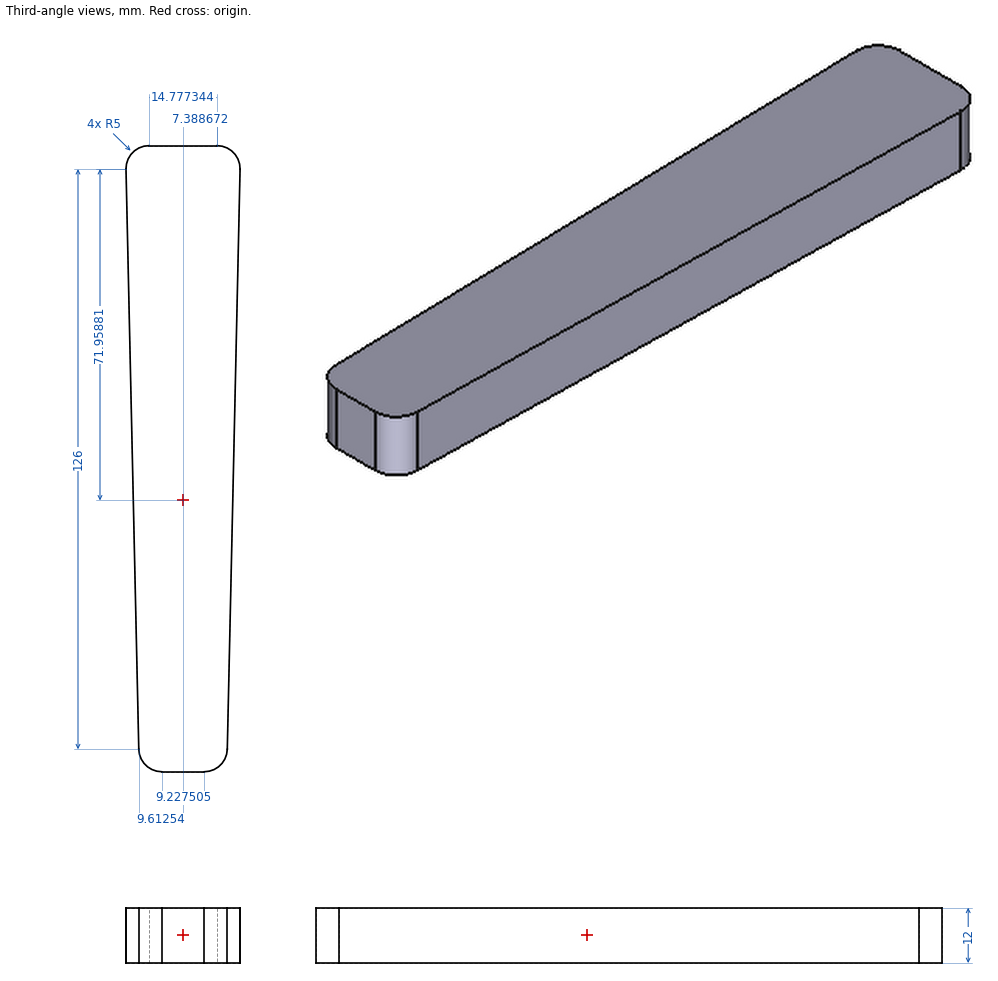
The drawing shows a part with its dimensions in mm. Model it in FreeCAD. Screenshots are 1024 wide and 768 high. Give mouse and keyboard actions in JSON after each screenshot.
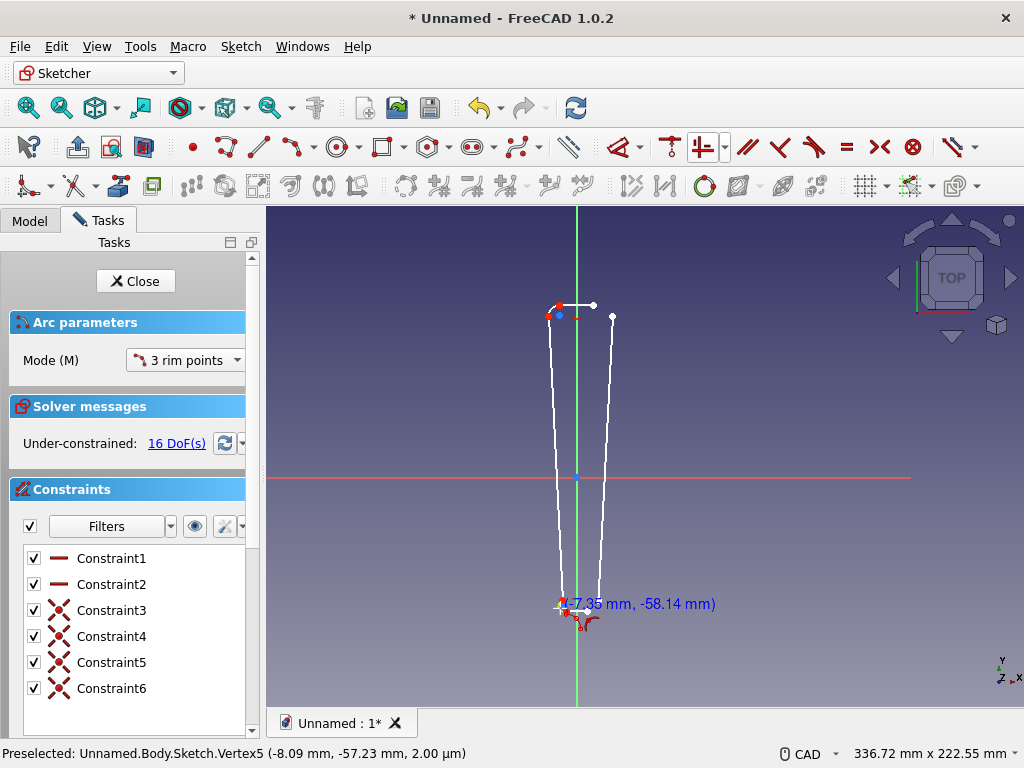
{"action": "scroll", "coordinate": [587, 611], "scroll_direction": "up", "scroll_amount": 3}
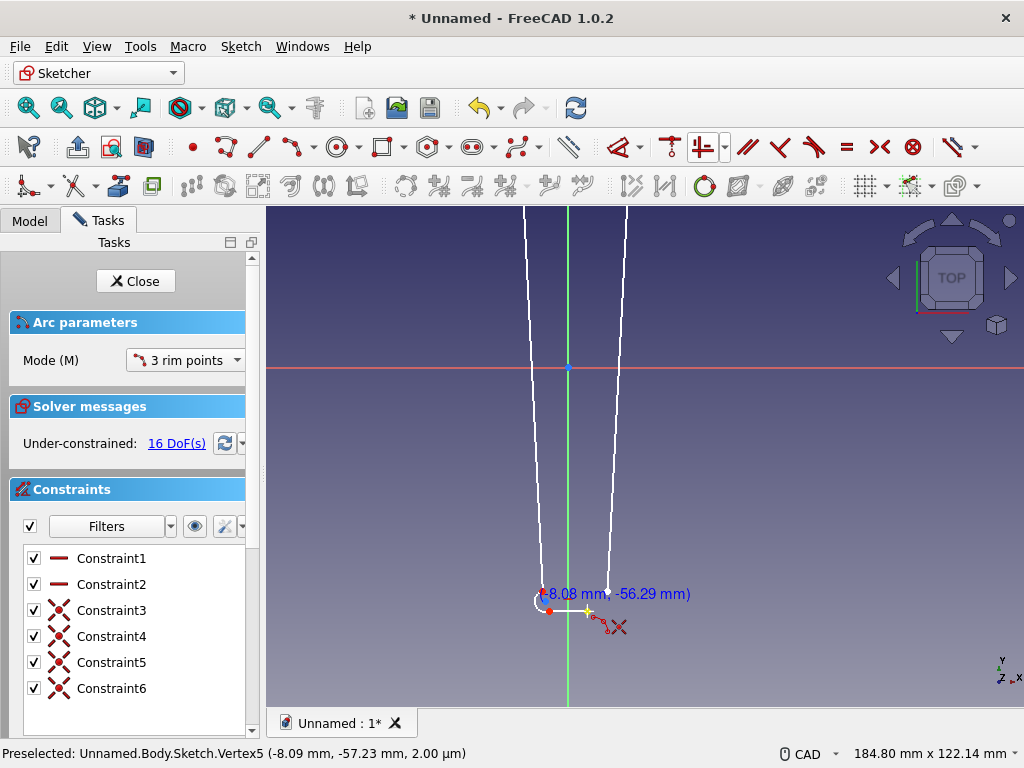
{"action": "left_click", "coordinate": [587, 611]}
{"action": "left_click", "coordinate": [607, 591]}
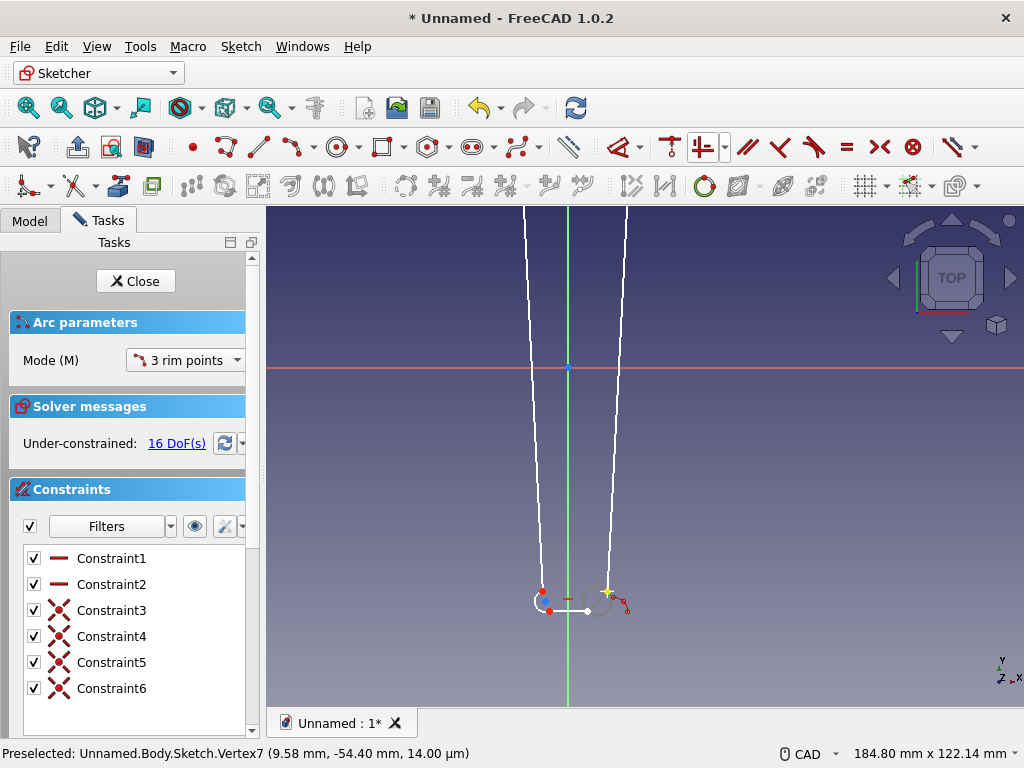
{"action": "scroll", "coordinate": [601, 604], "scroll_direction": "up", "scroll_amount": 5}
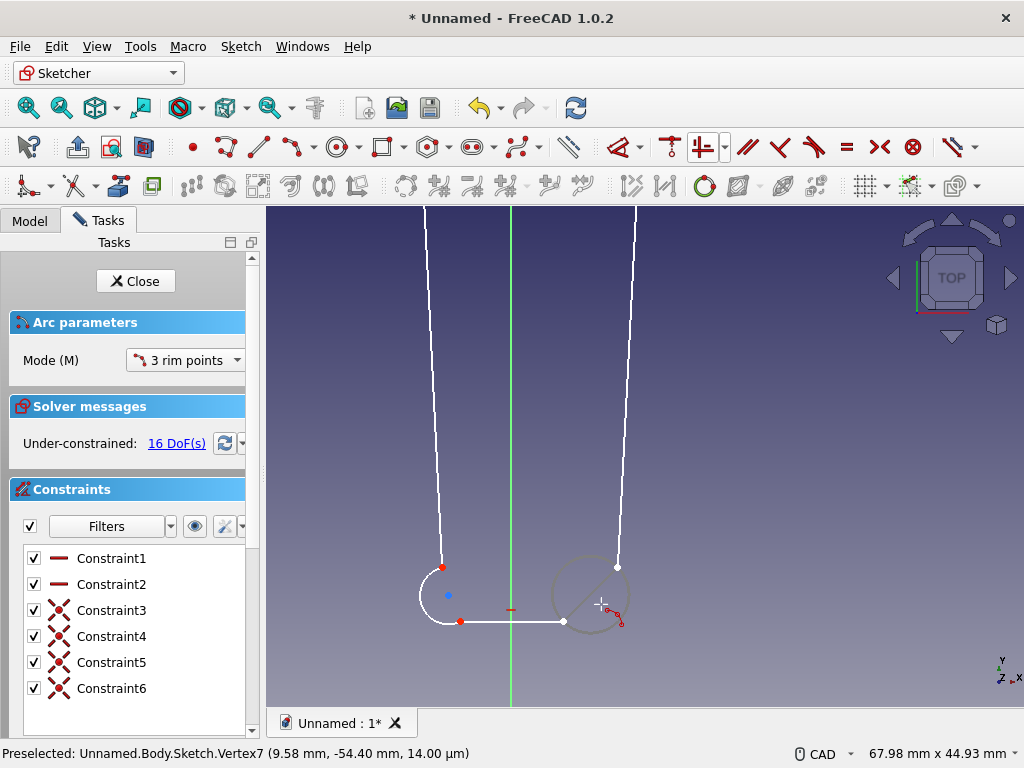
{"action": "left_click", "coordinate": [601, 602]}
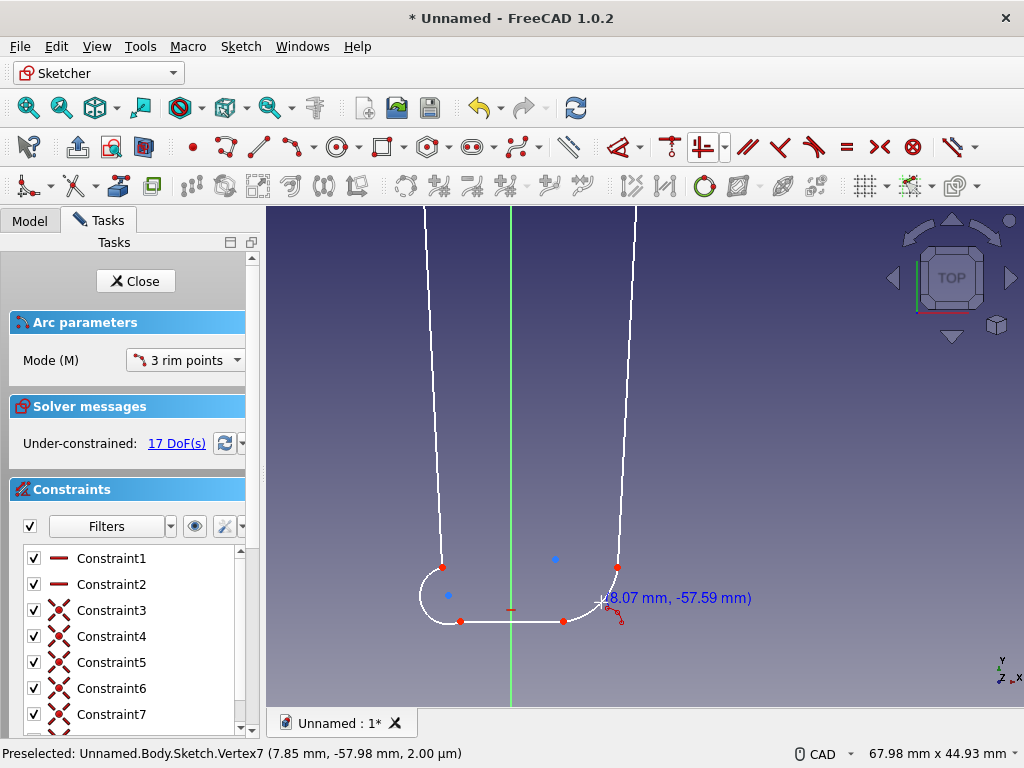
{"action": "scroll", "coordinate": [593, 607], "scroll_direction": "down", "scroll_amount": 8}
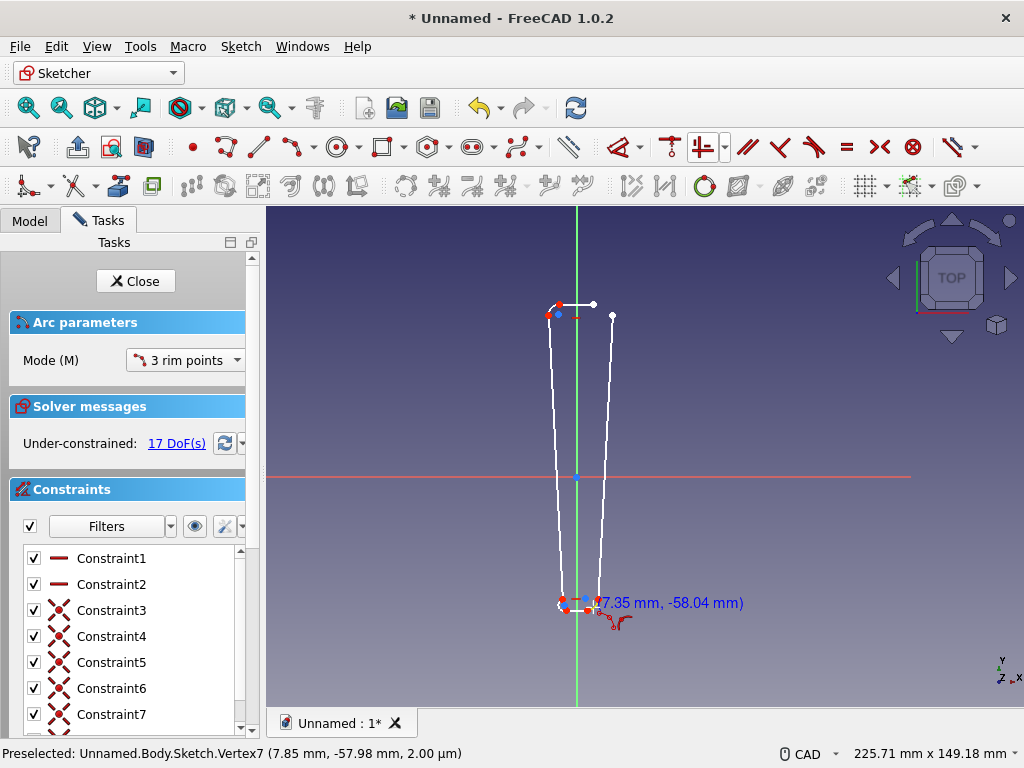
{"action": "left_click", "coordinate": [613, 316]}
{"action": "left_click", "coordinate": [594, 305]}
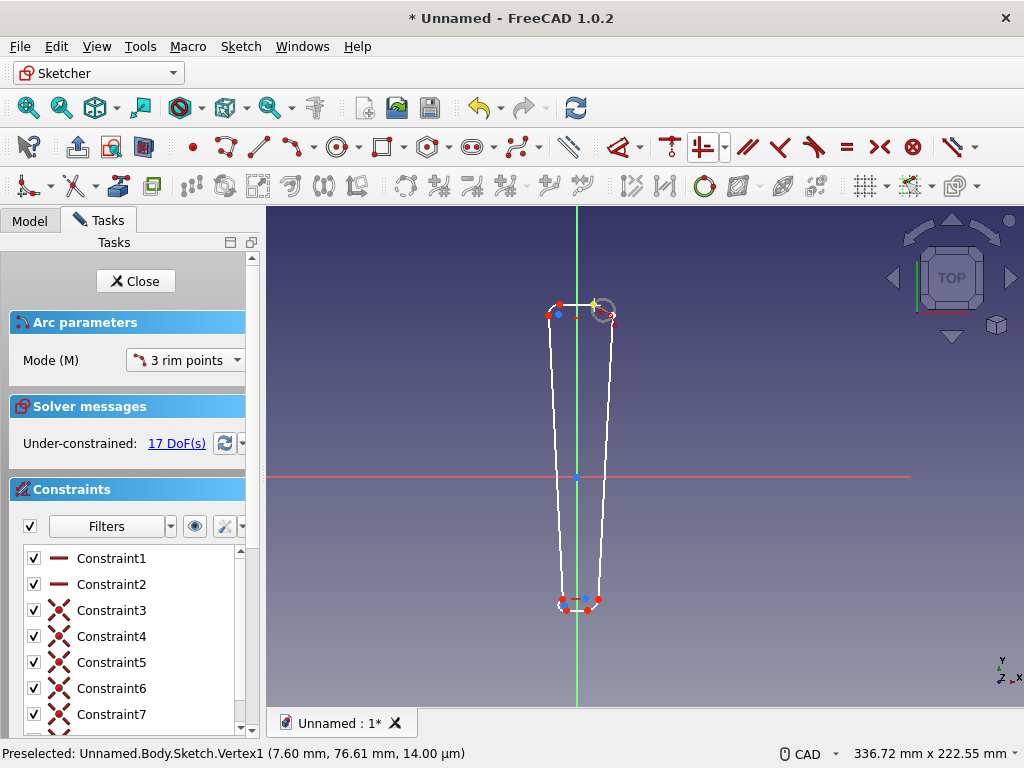
{"action": "scroll", "coordinate": [601, 307], "scroll_direction": "up", "scroll_amount": 8}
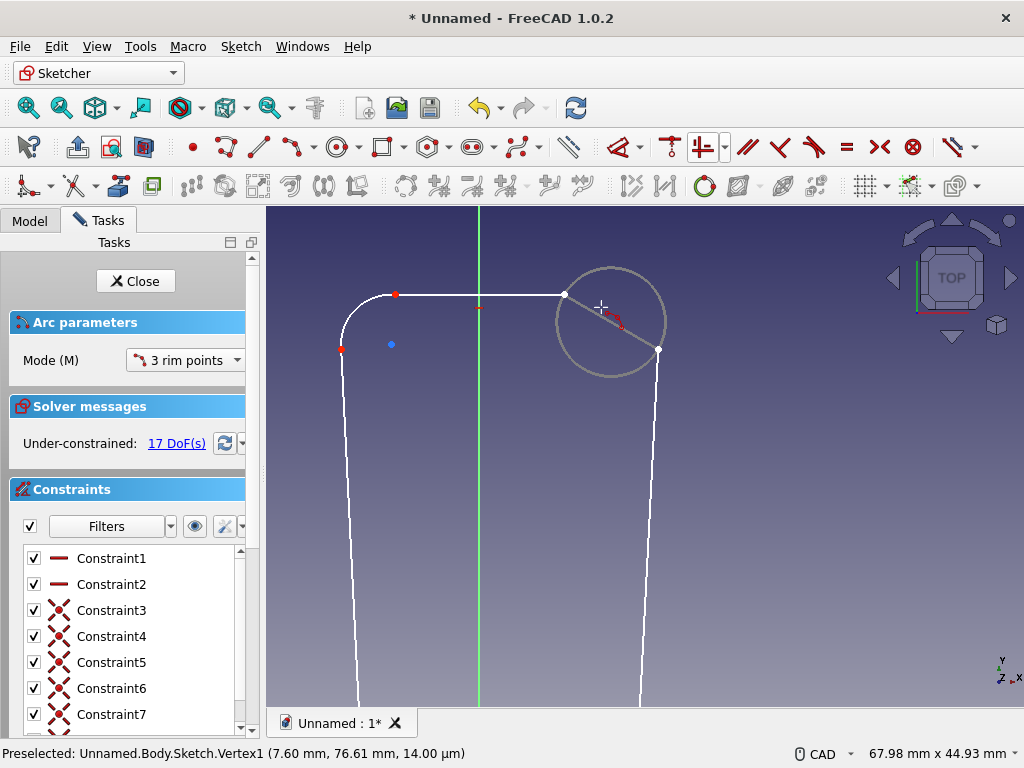
{"action": "left_click", "coordinate": [602, 307]}
{"action": "key", "text": "Escape"}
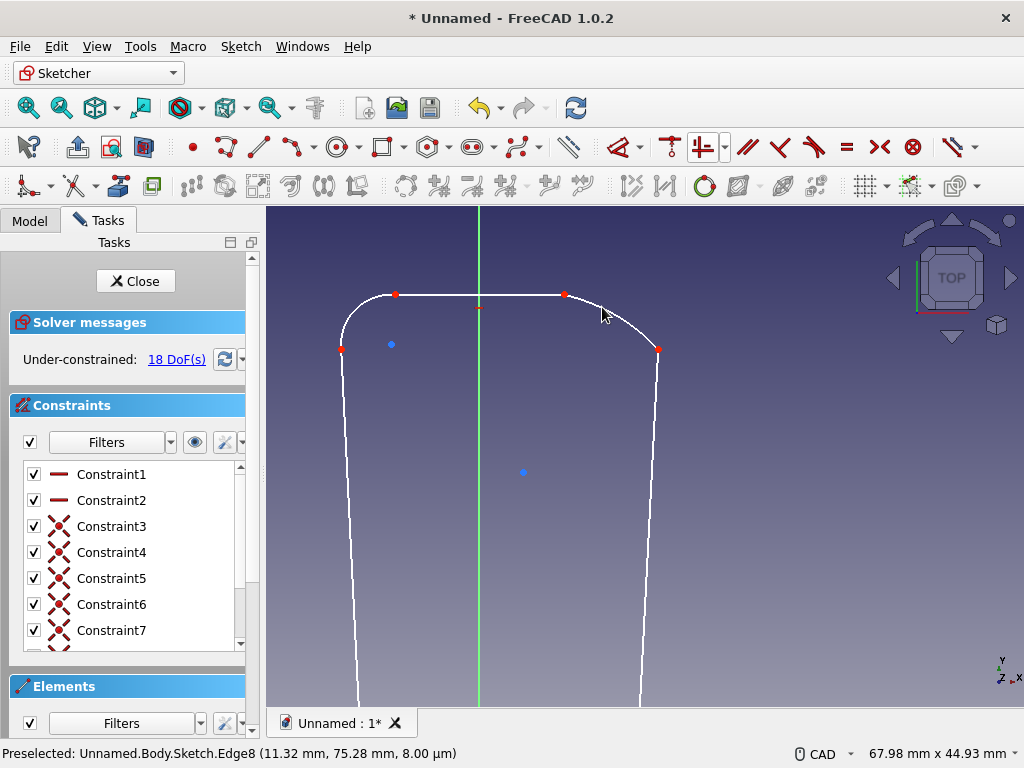
{"action": "left_click", "coordinate": [514, 295]}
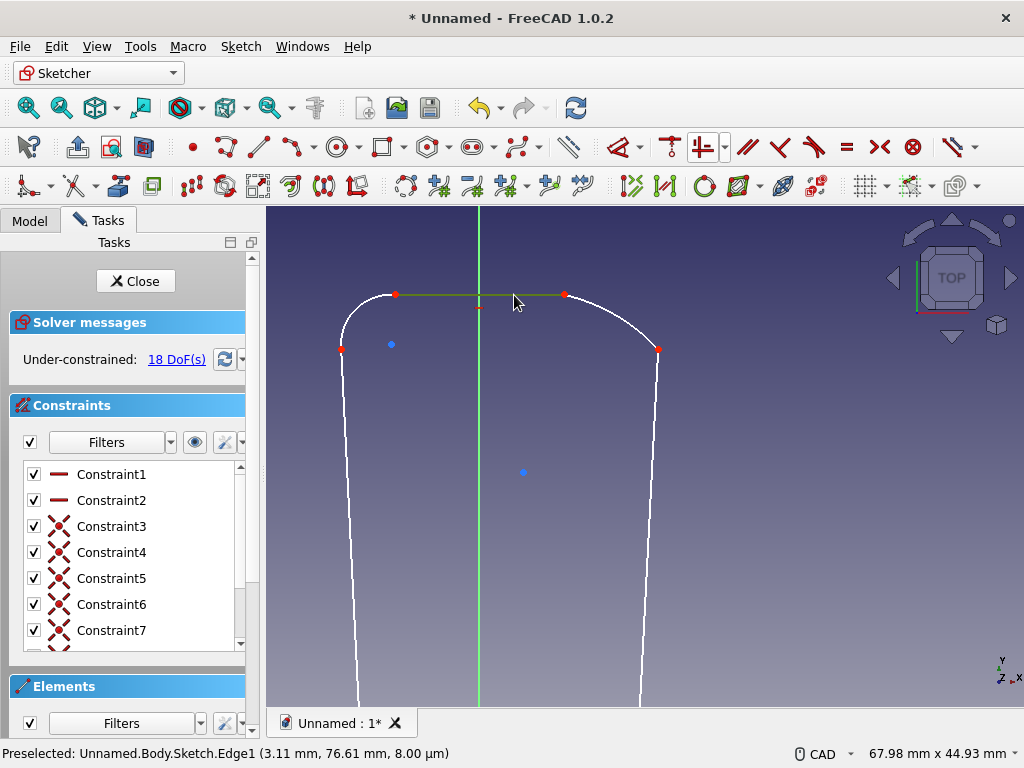
{"action": "left_click", "coordinate": [370, 299]}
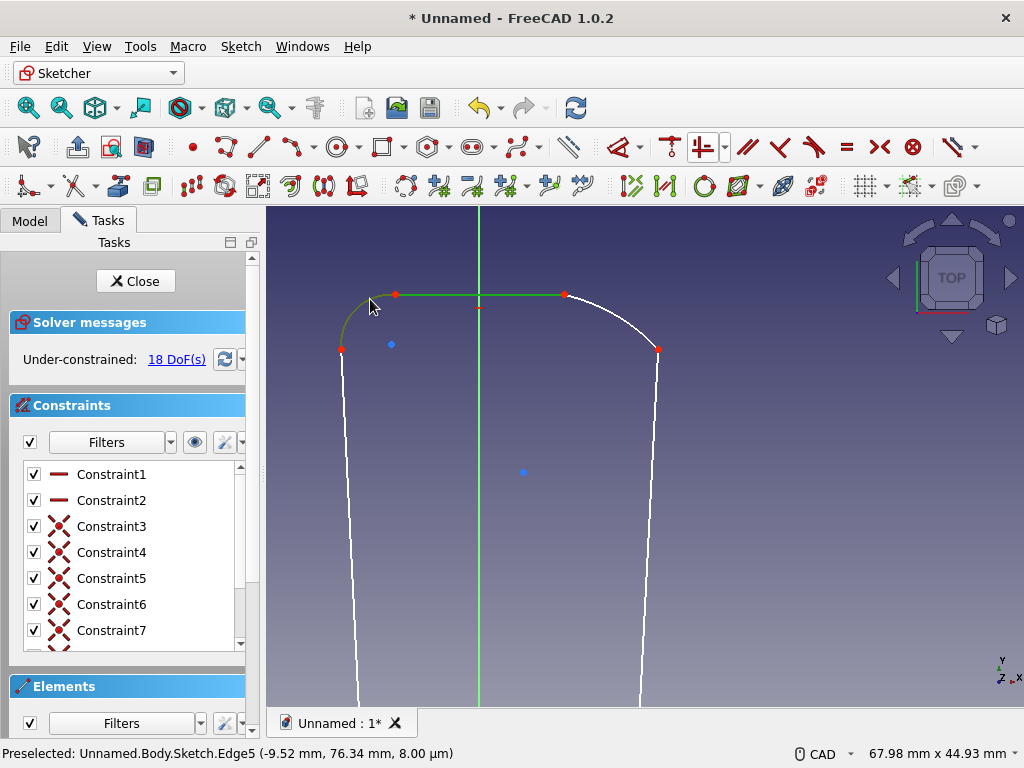
{"action": "key", "text": "t"}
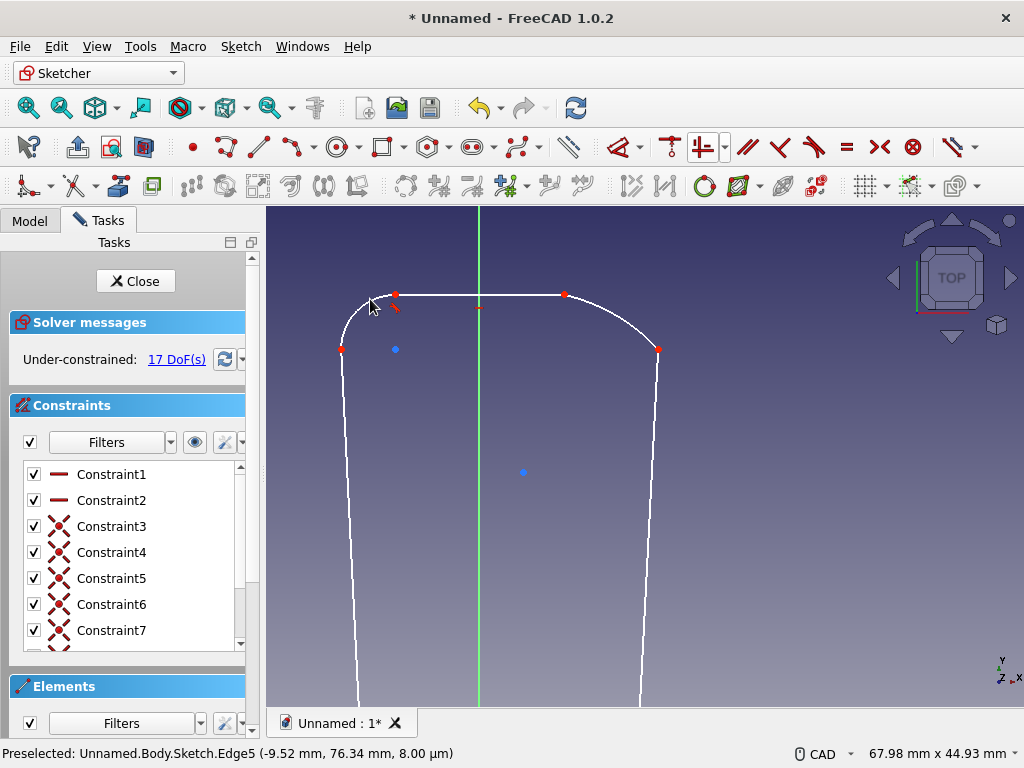
{"action": "left_click", "coordinate": [514, 295]}